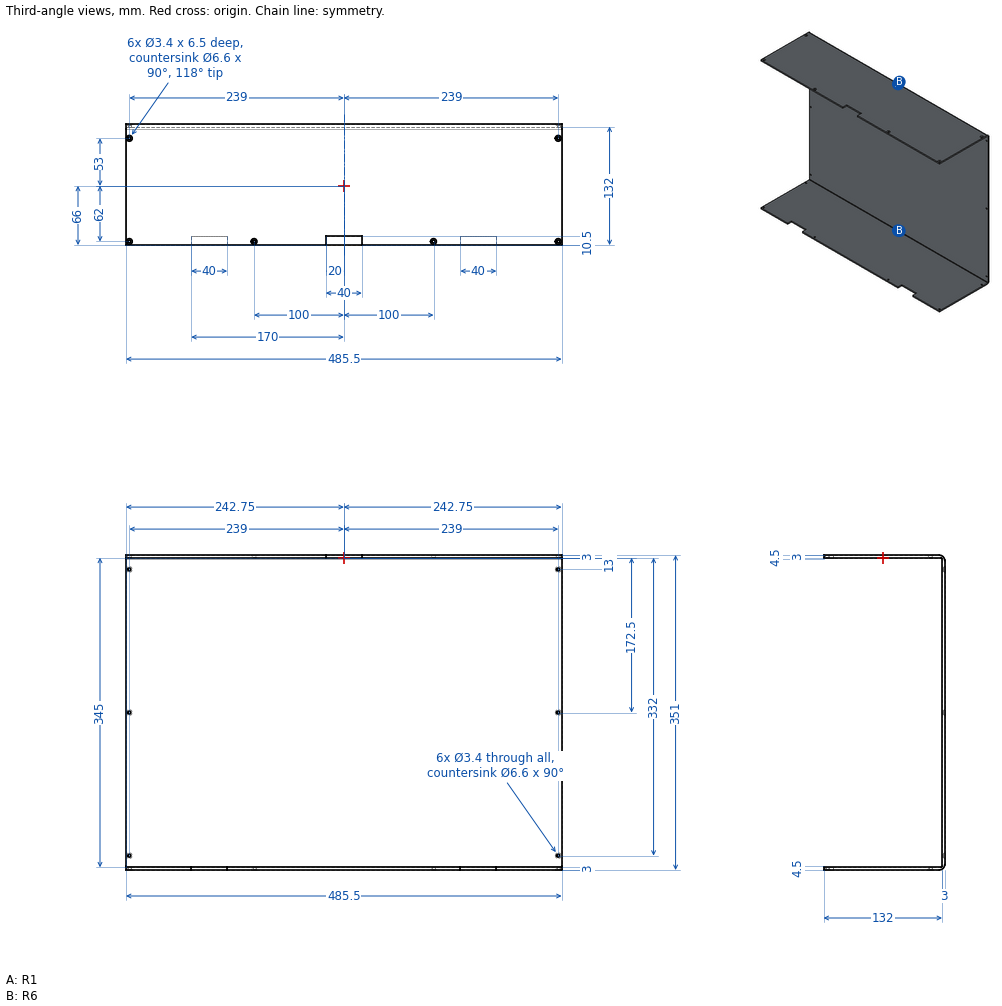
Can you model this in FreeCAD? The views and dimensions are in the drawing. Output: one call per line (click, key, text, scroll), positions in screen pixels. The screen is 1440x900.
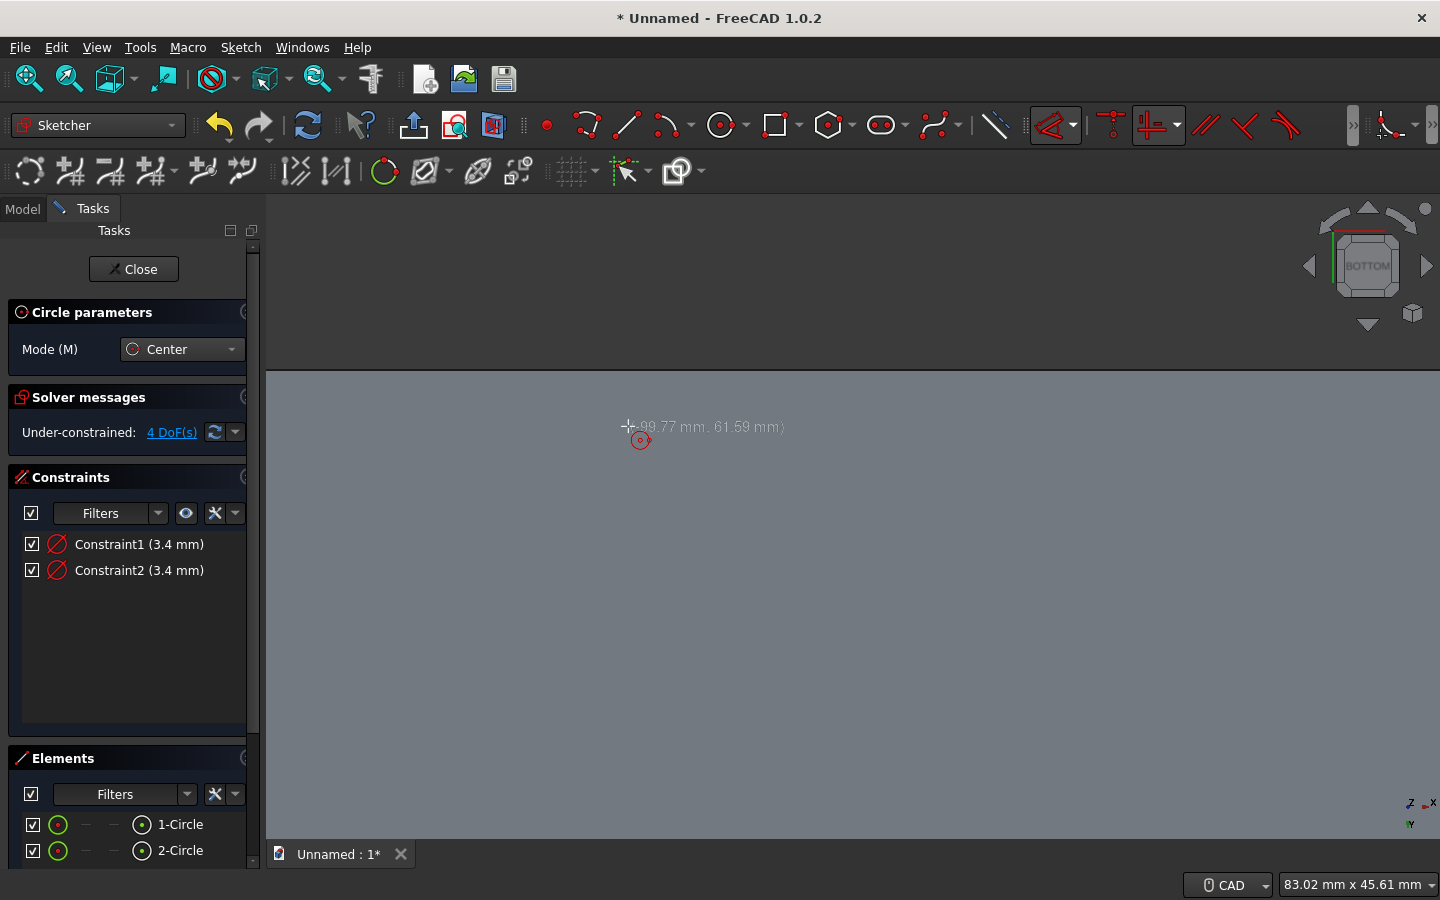
scroll(628, 426, down, 11)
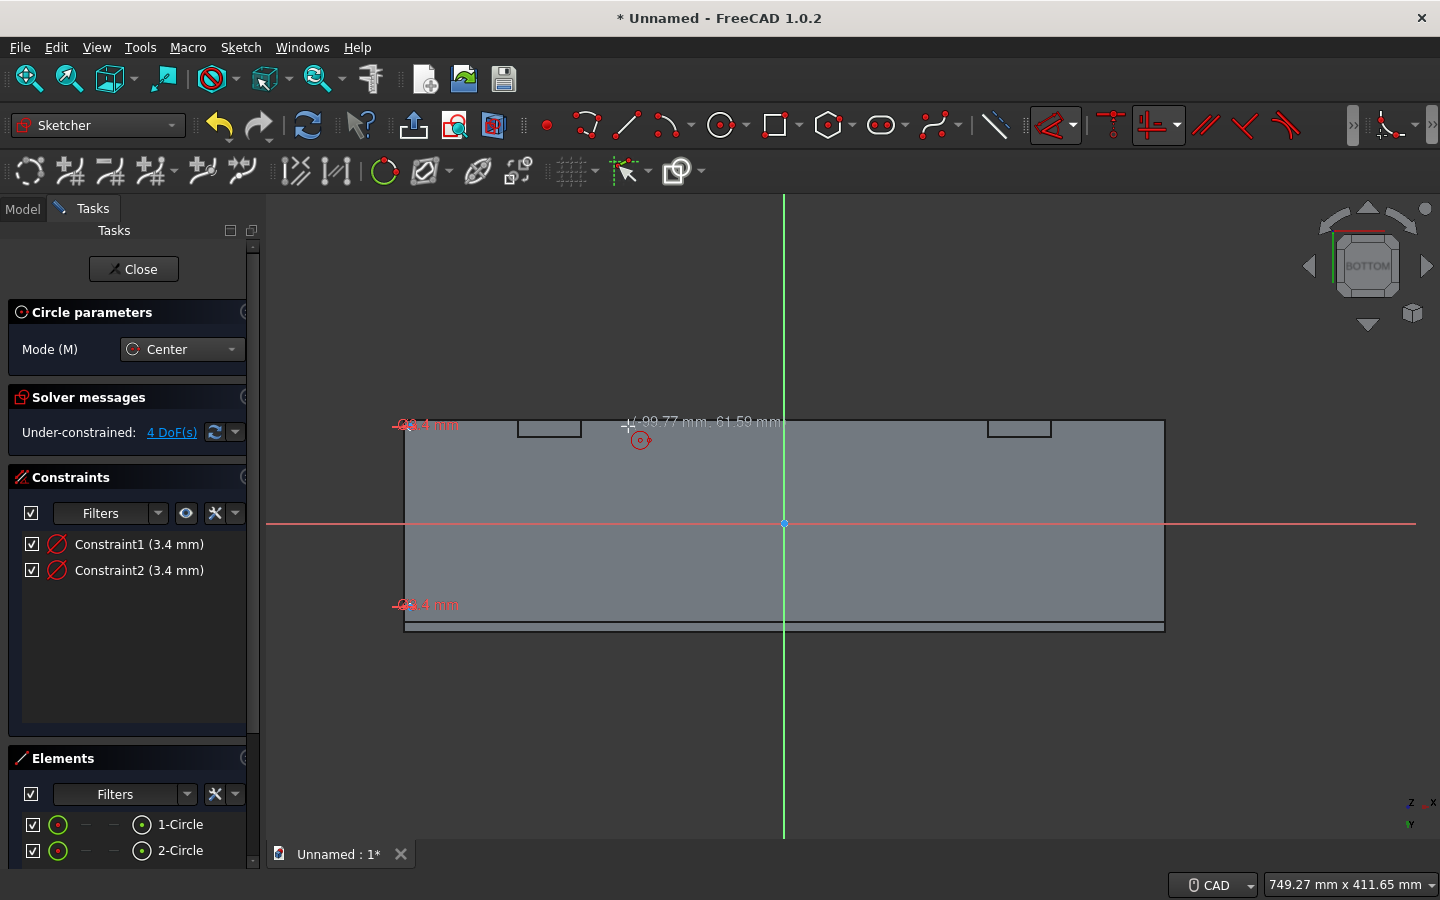
click(628, 426)
move(630, 424)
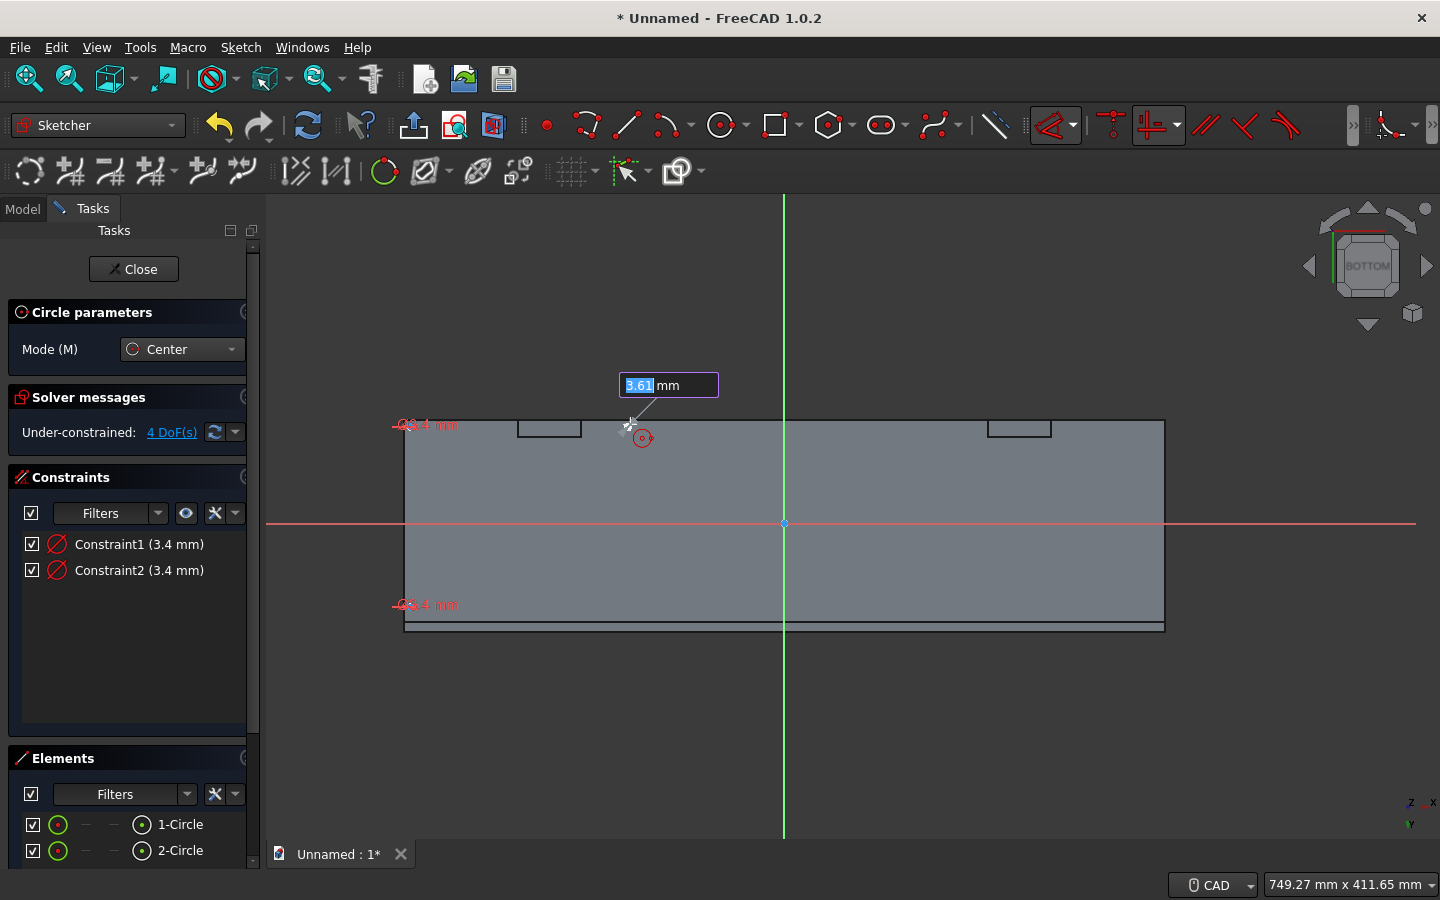
text(3.4)
key(Return)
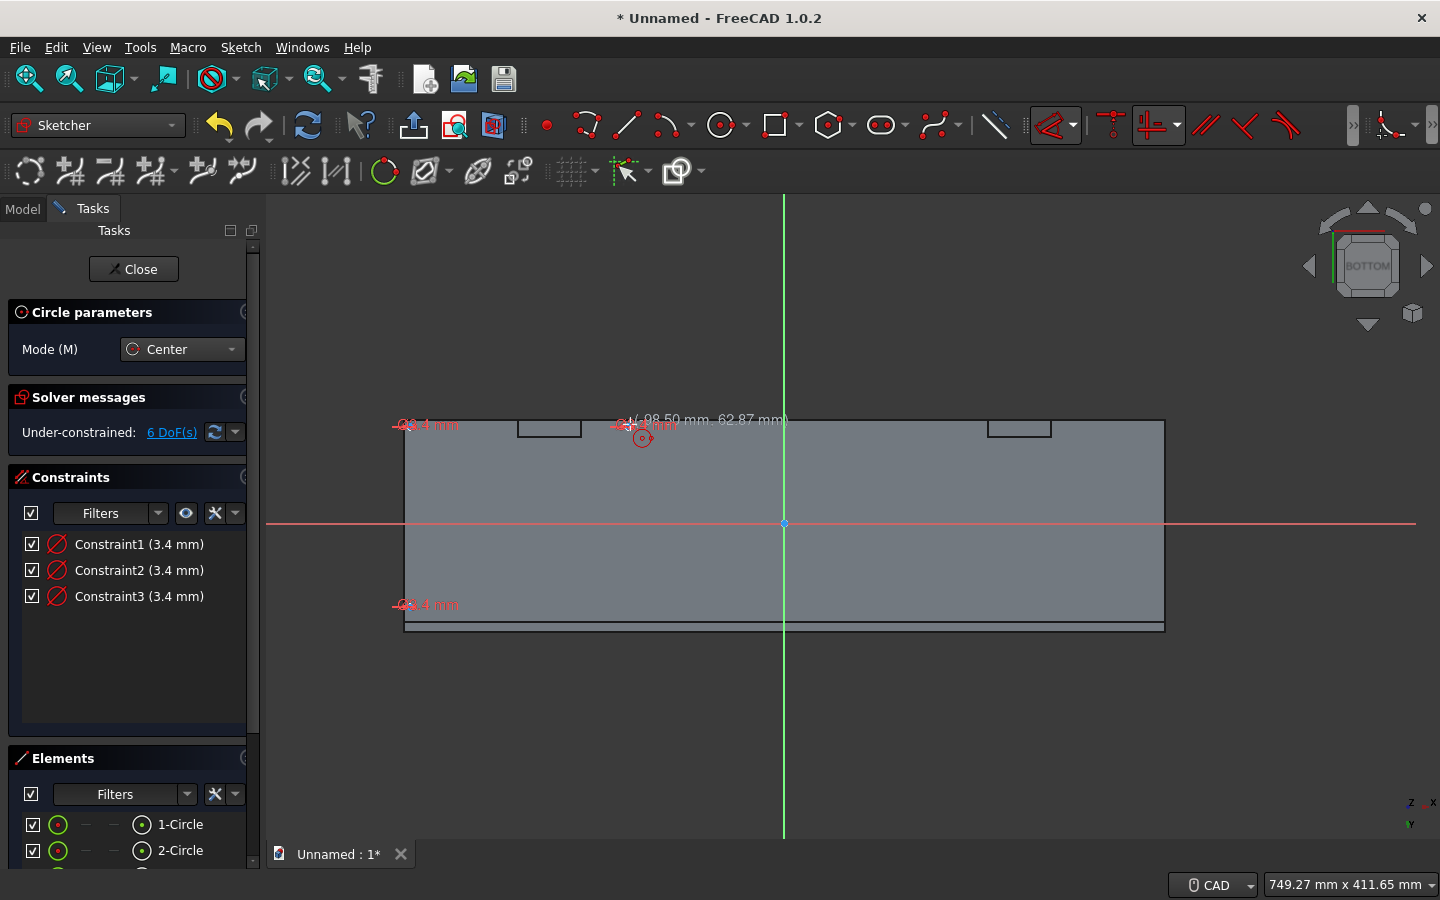
scroll(941, 426, up, 11)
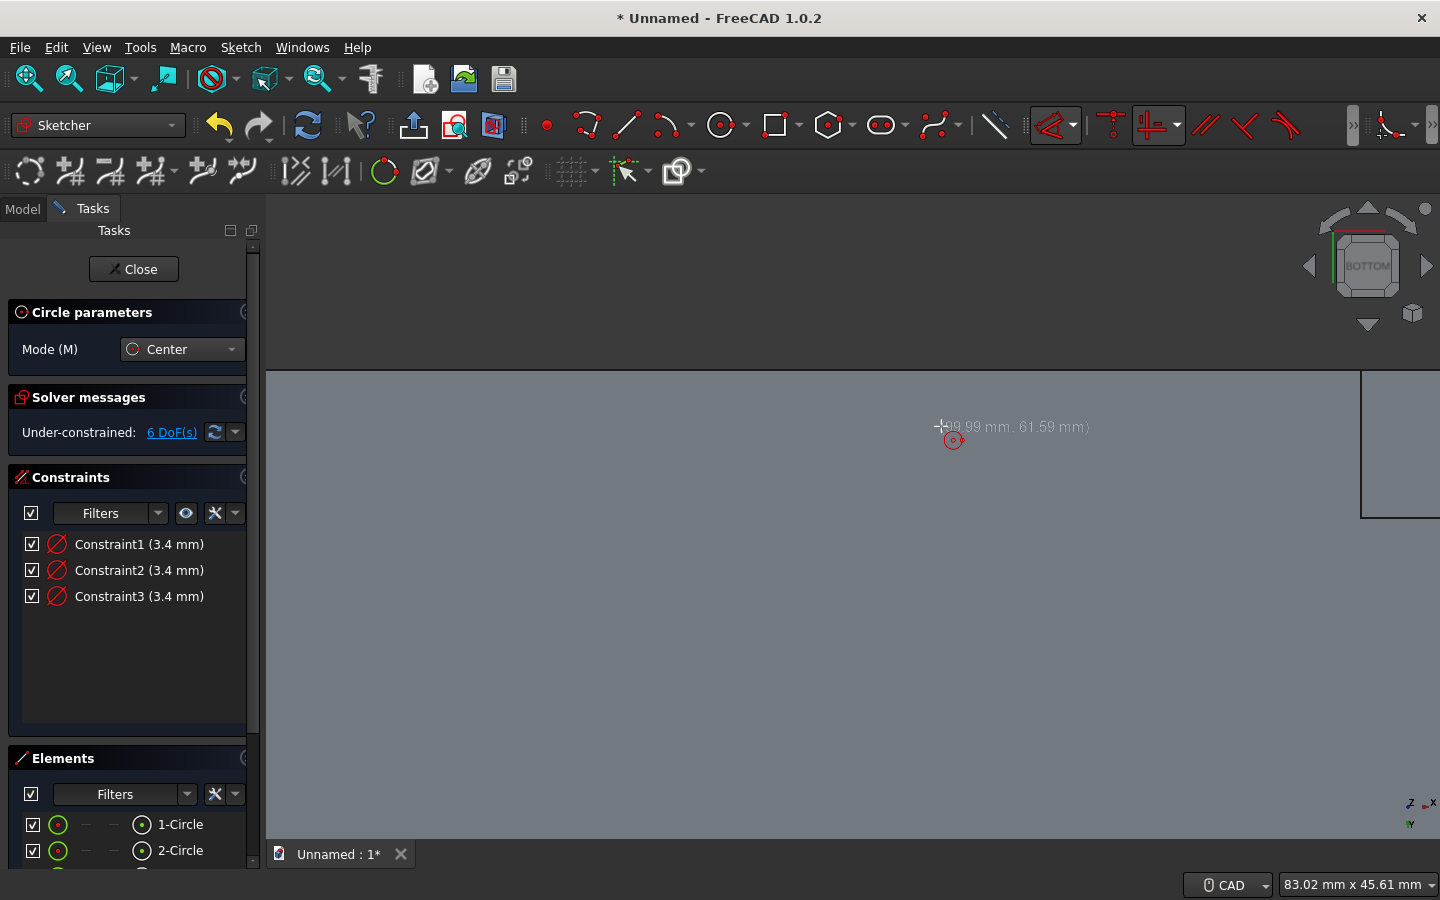
scroll(942, 426, down, 11)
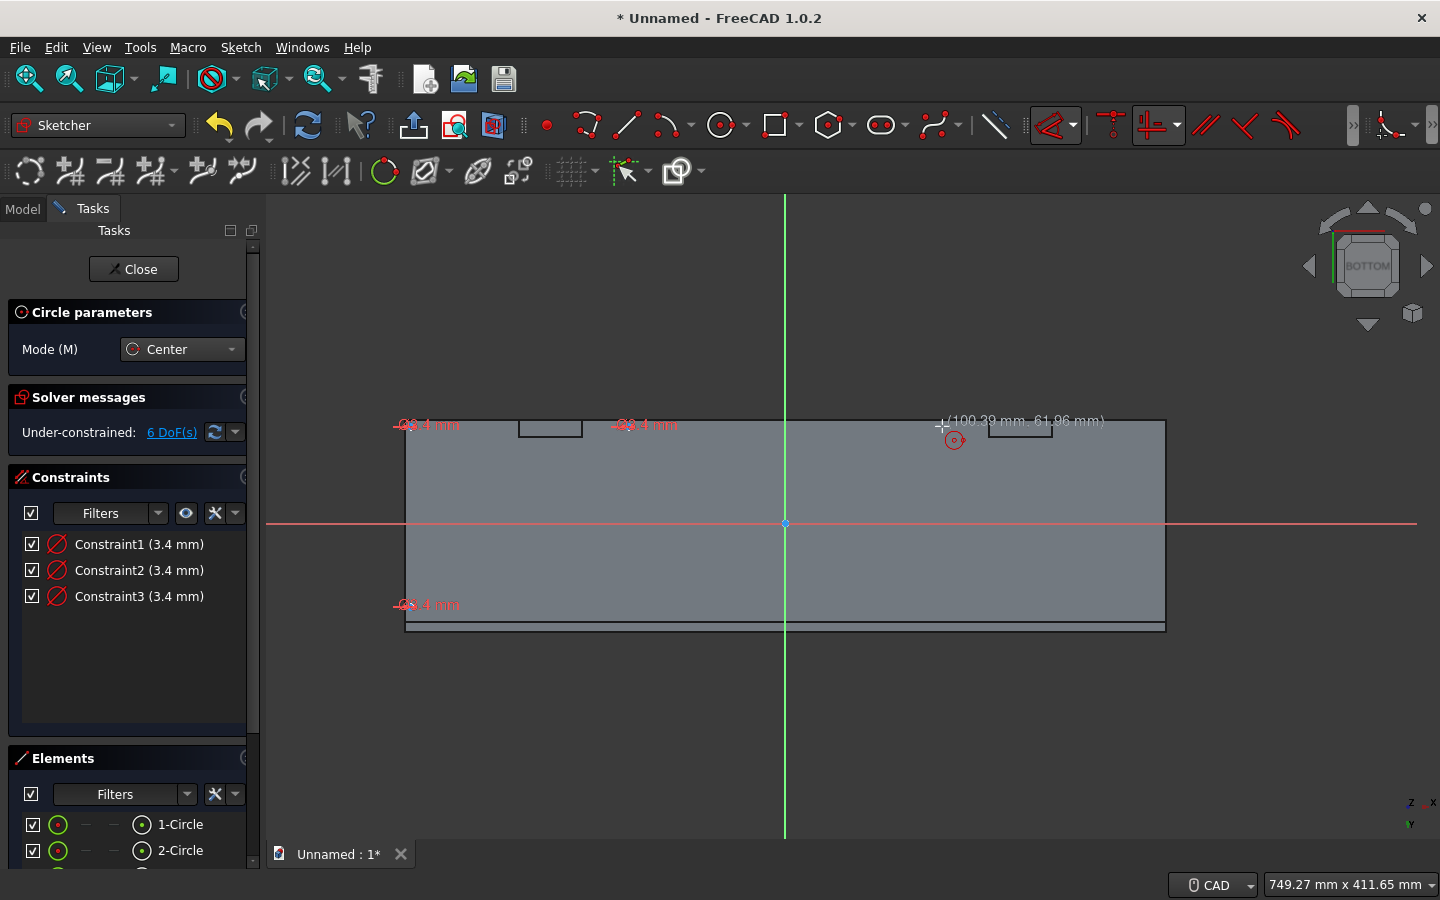
click(942, 426)
move(944, 424)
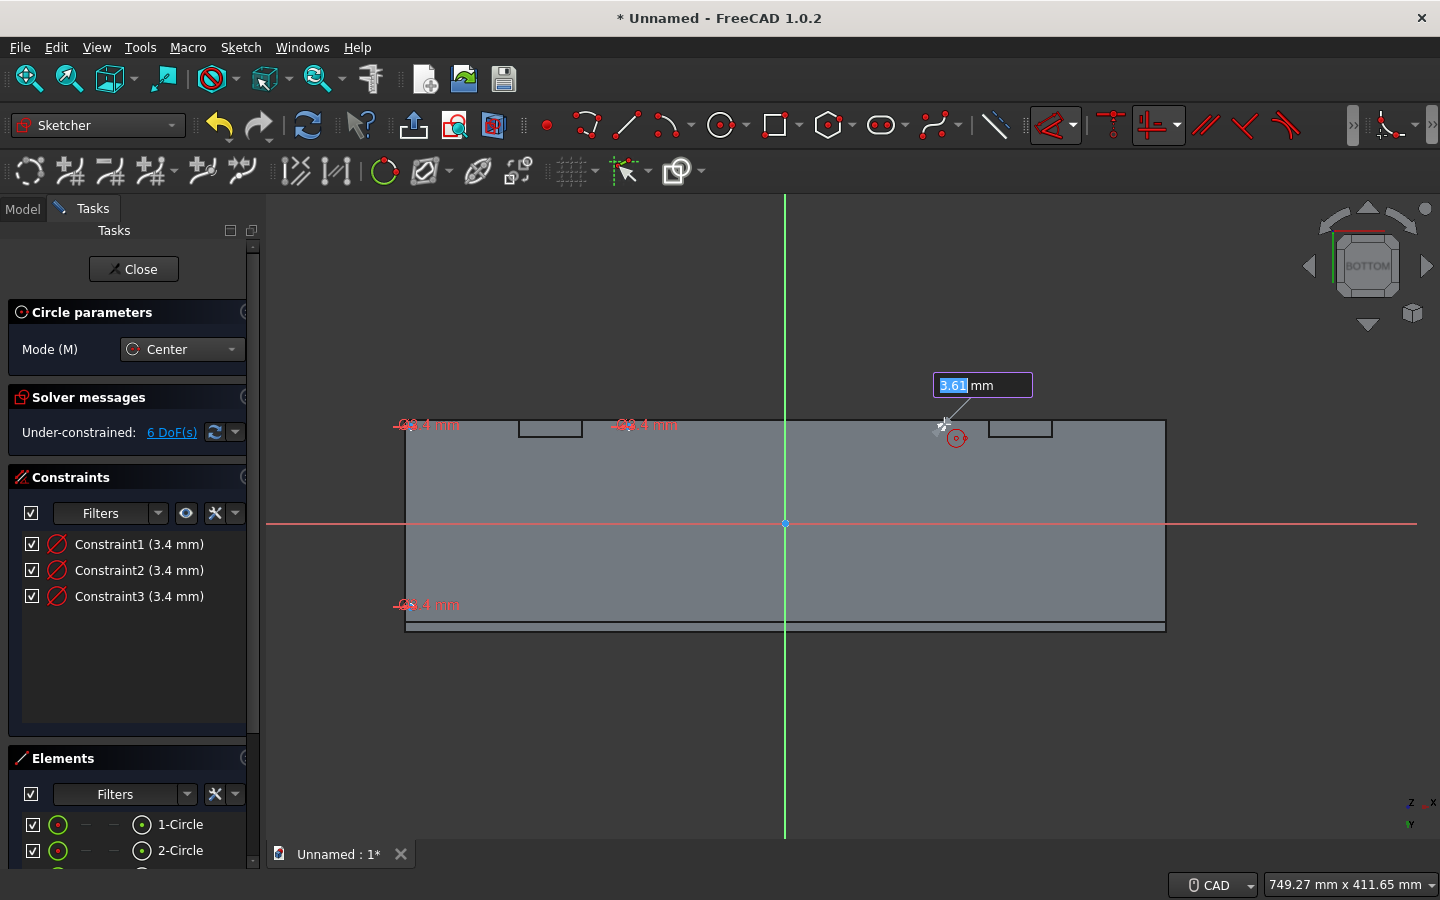
text(3.4)
key(Return)